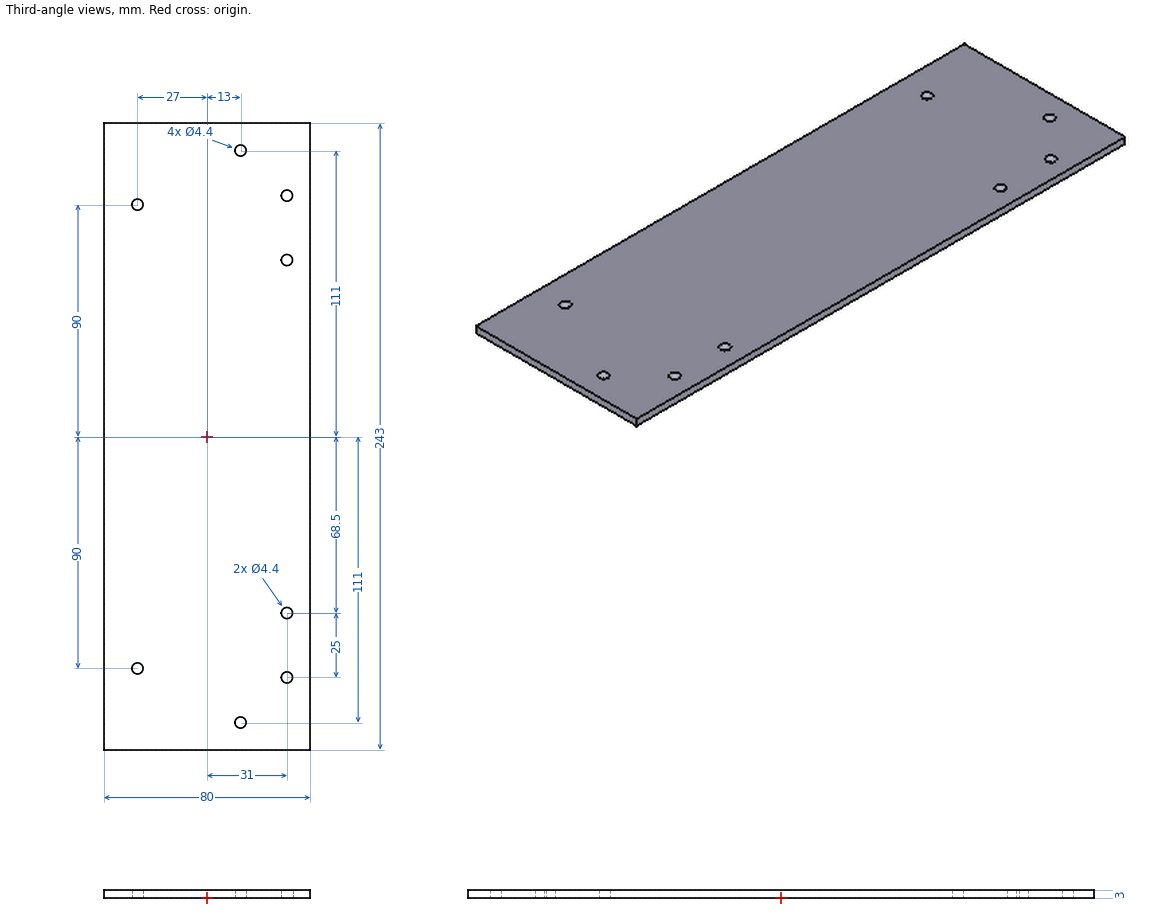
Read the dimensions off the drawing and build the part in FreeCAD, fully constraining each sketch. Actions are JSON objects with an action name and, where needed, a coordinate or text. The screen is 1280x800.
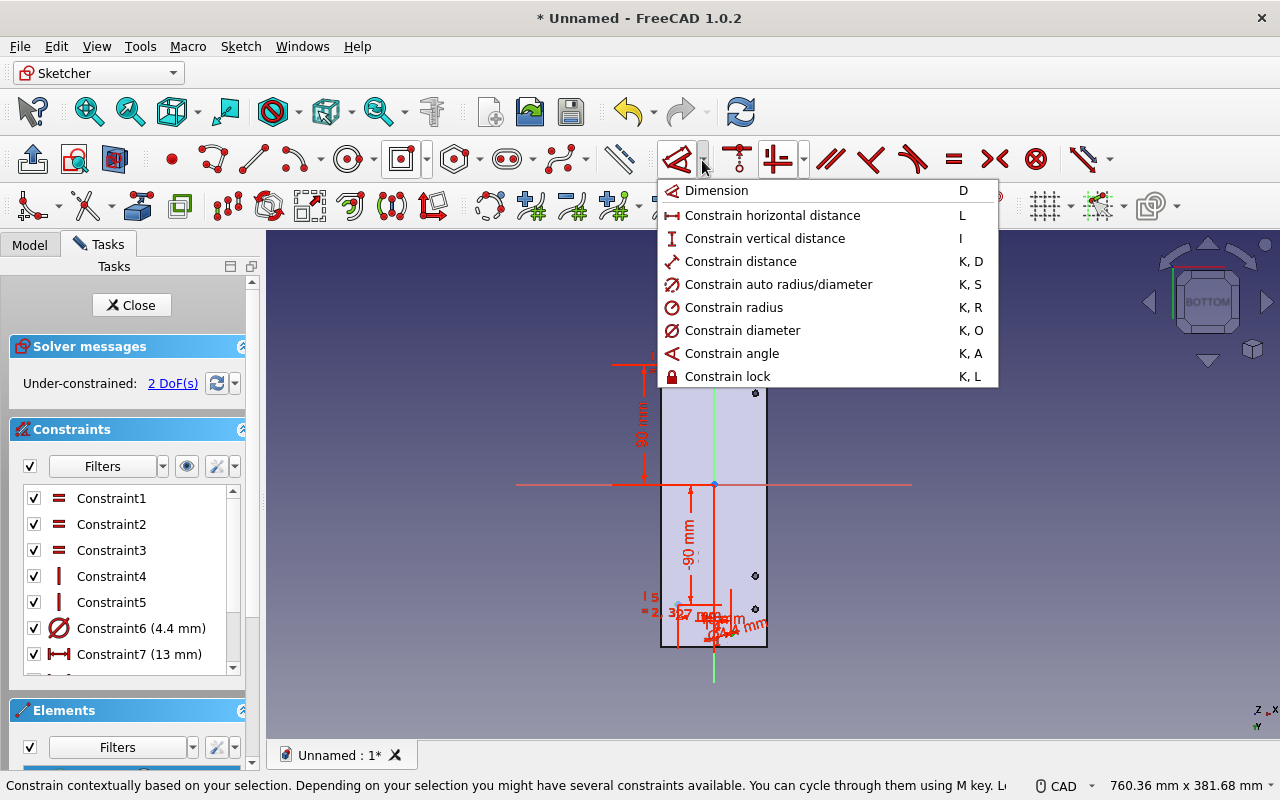
{"action": "left_click", "coordinate": [828, 238]}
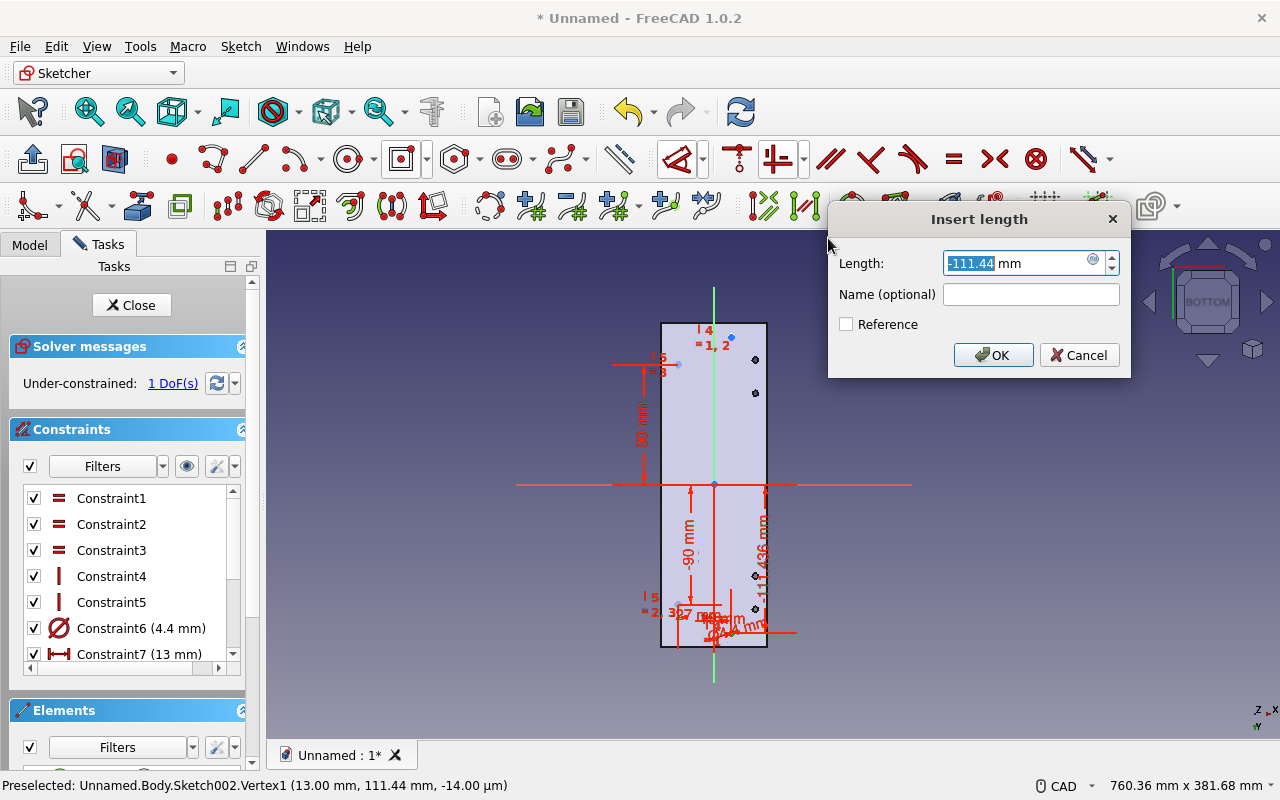
{"action": "type", "text": "-111"}
{"action": "key", "text": "Return"}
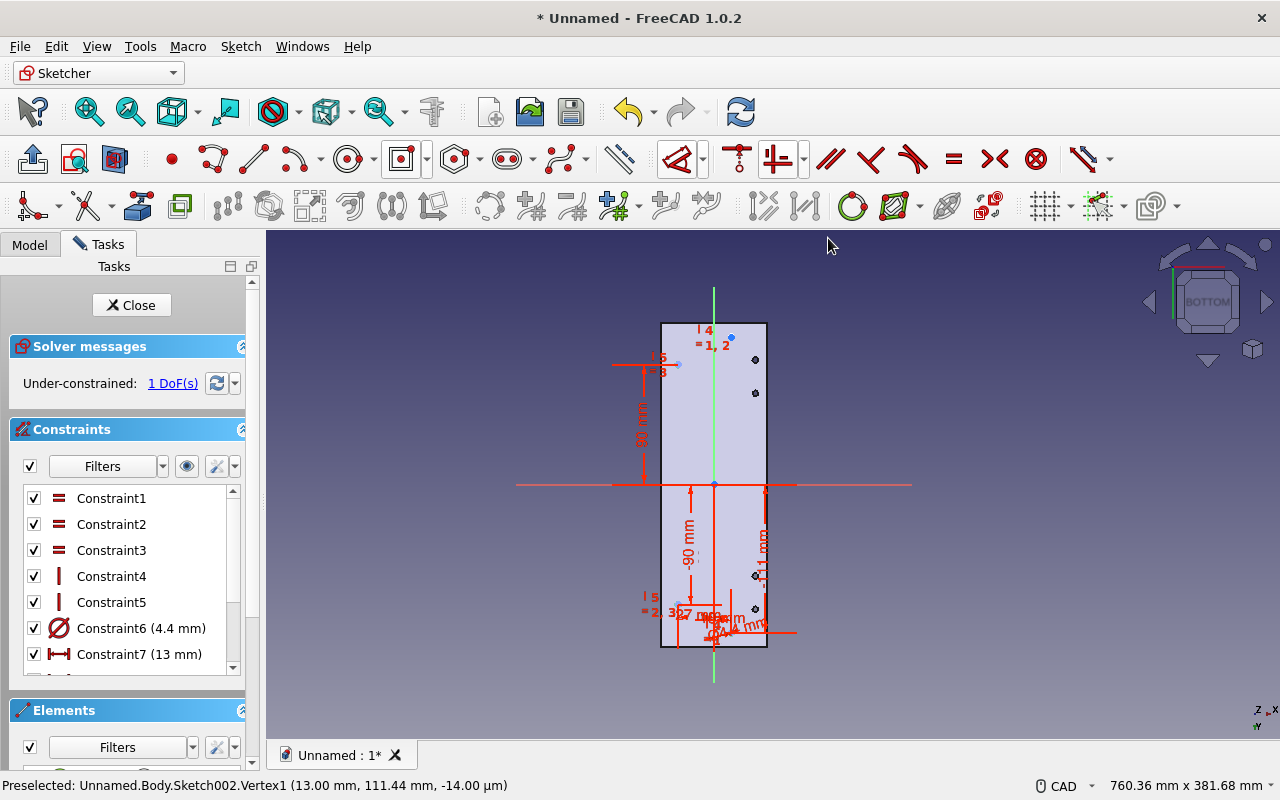
{"action": "left_click", "coordinate": [731, 337]}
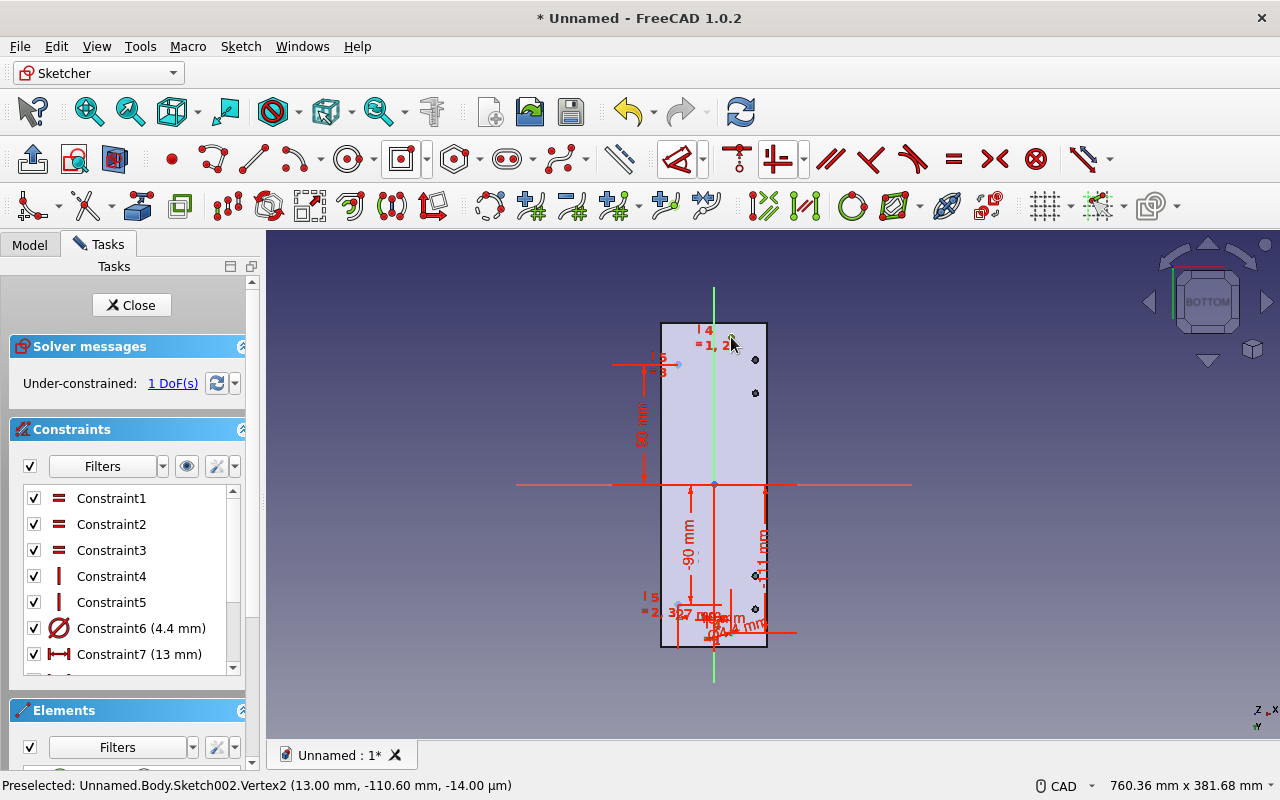
{"action": "left_click", "coordinate": [702, 160]}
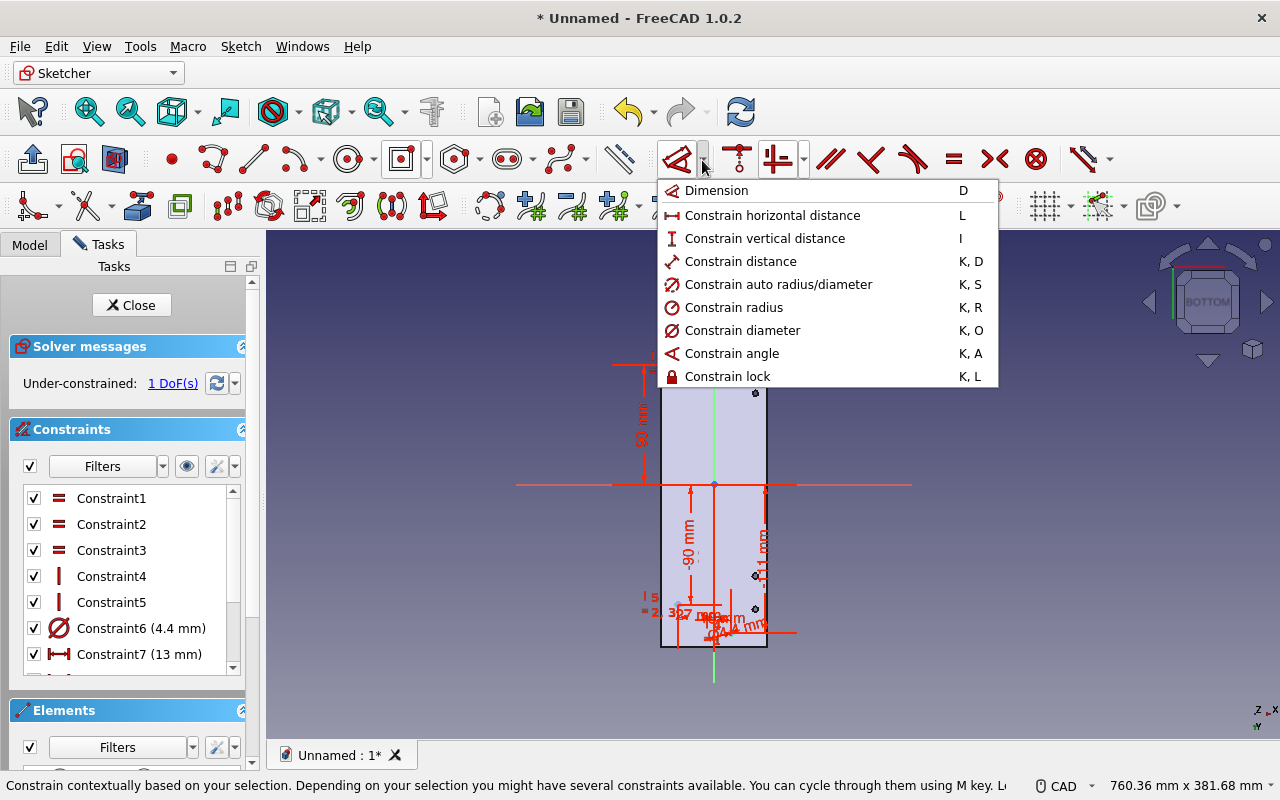
{"action": "left_click", "coordinate": [828, 238]}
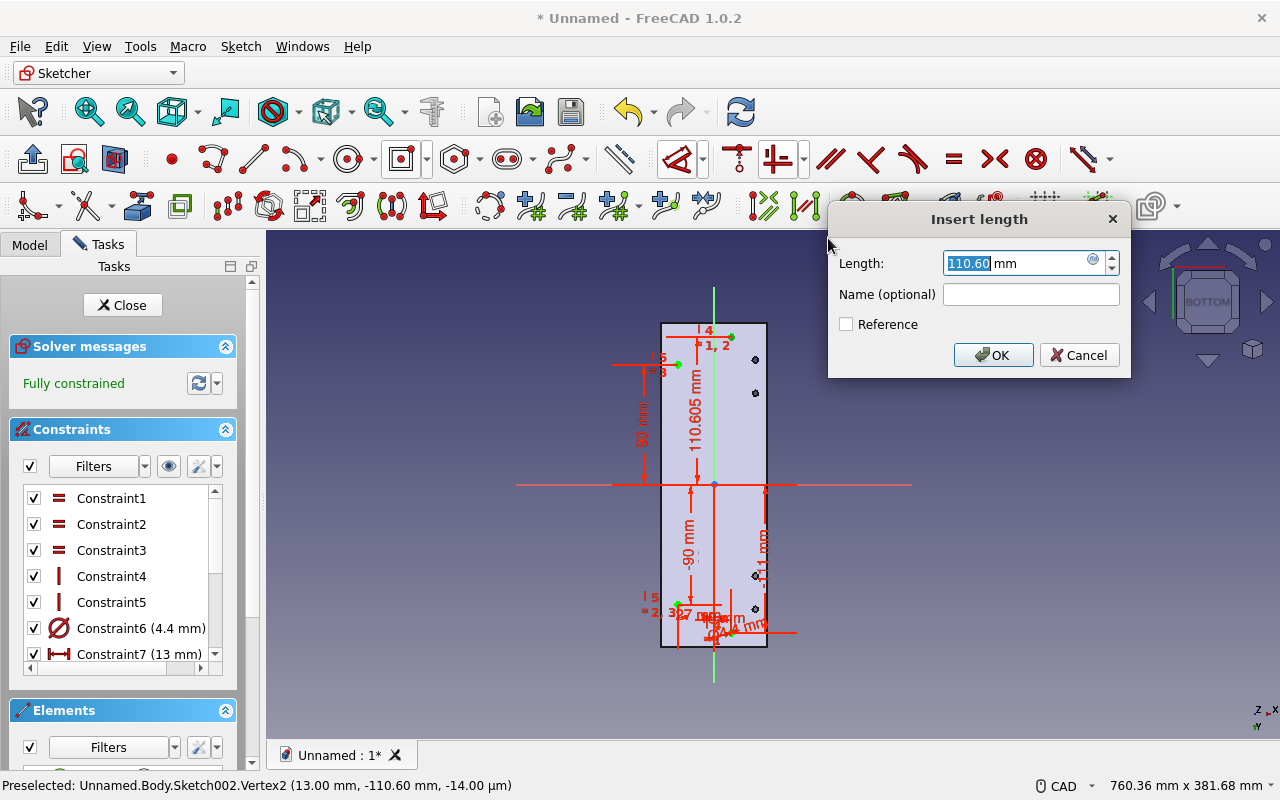
{"action": "type", "text": "111"}
{"action": "key", "text": "Return"}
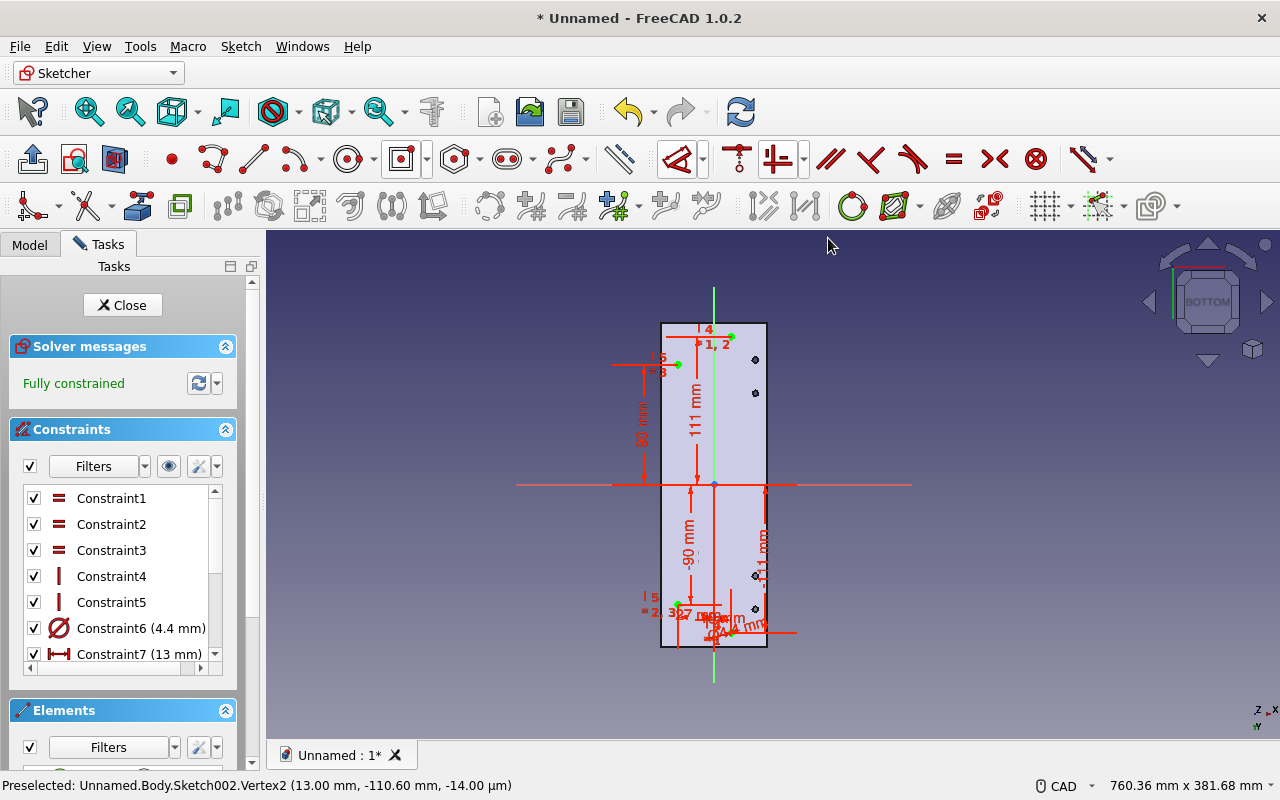
{"action": "left_click", "coordinate": [123, 305]}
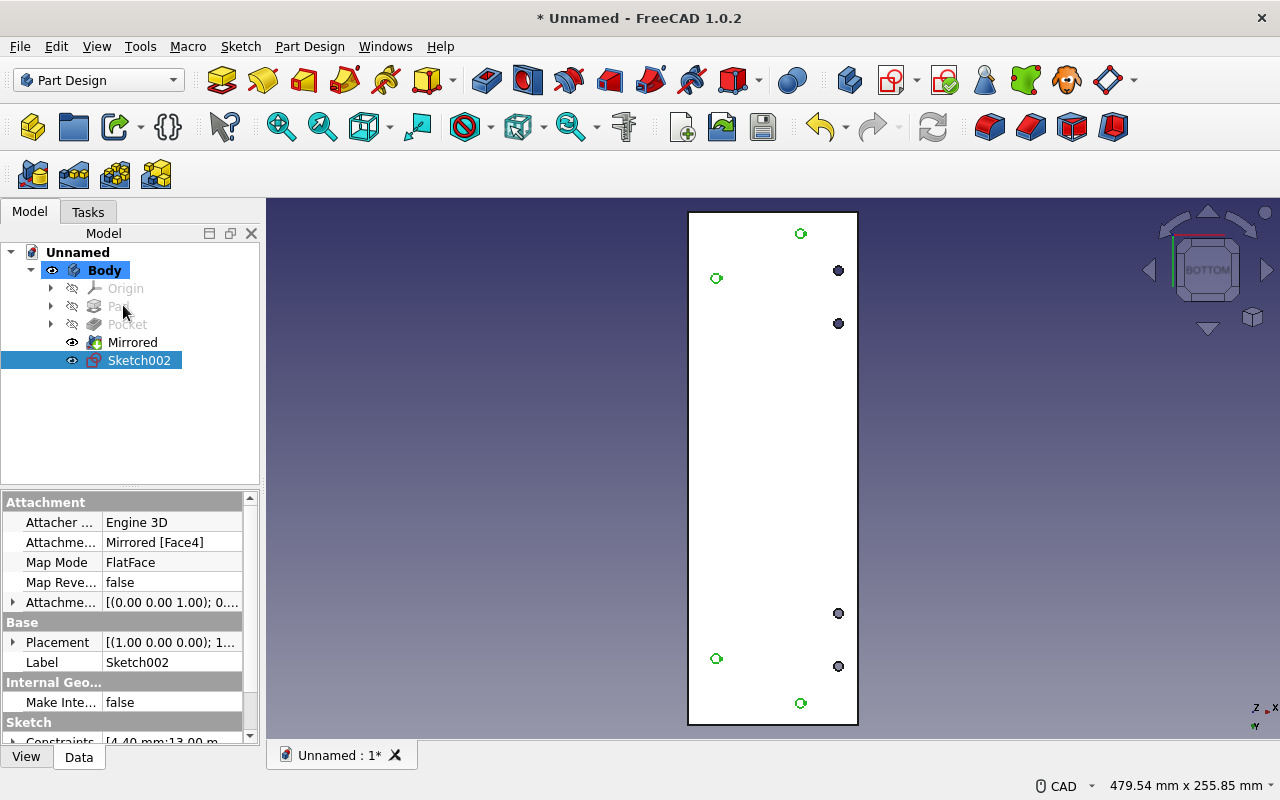
{"action": "left_click", "coordinate": [487, 80]}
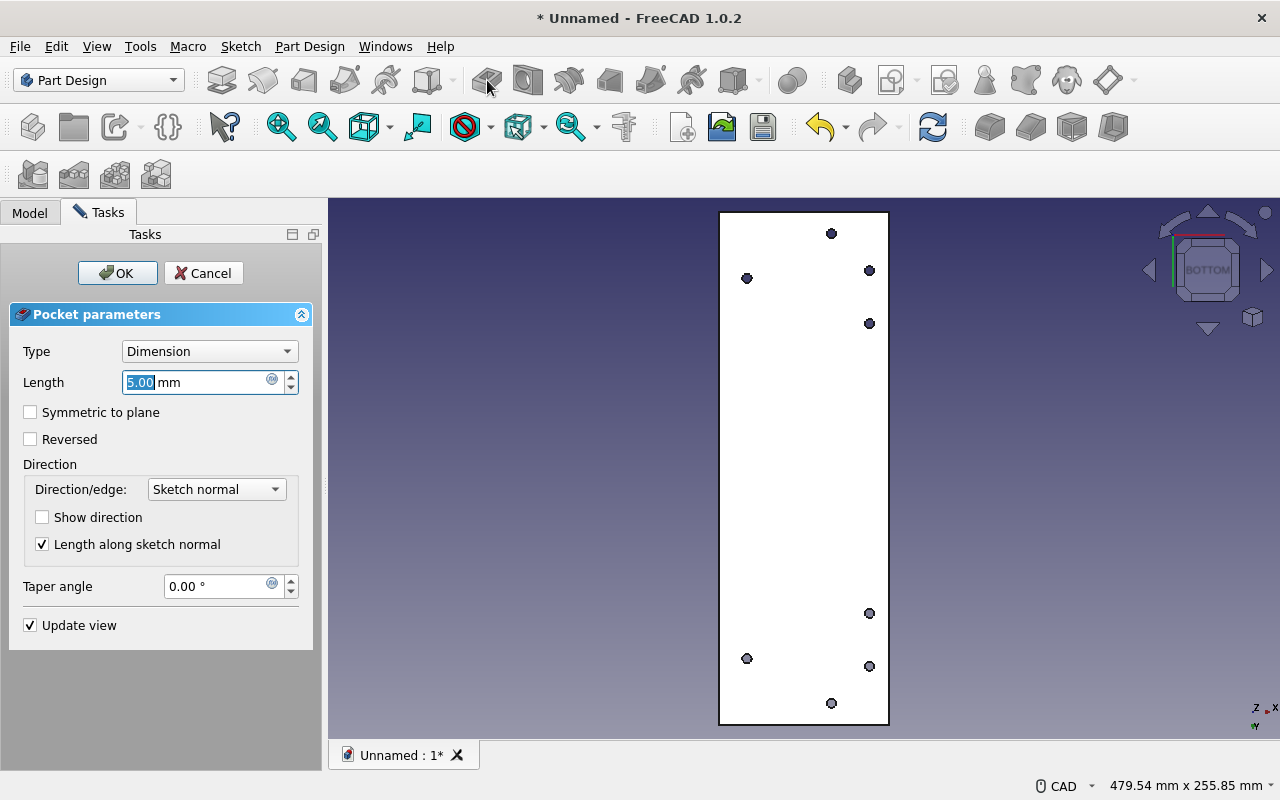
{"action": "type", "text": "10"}
{"action": "key", "text": "Tab"}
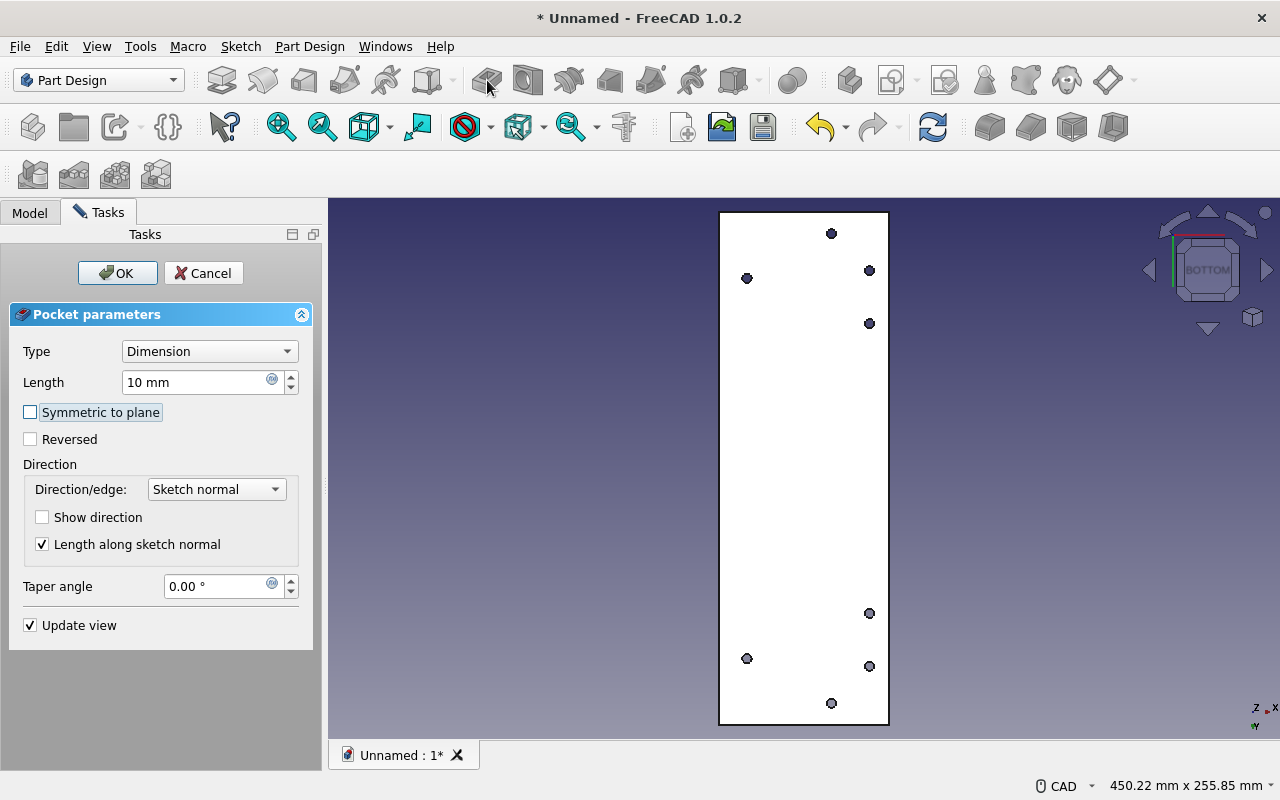
{"action": "left_click", "coordinate": [118, 273]}